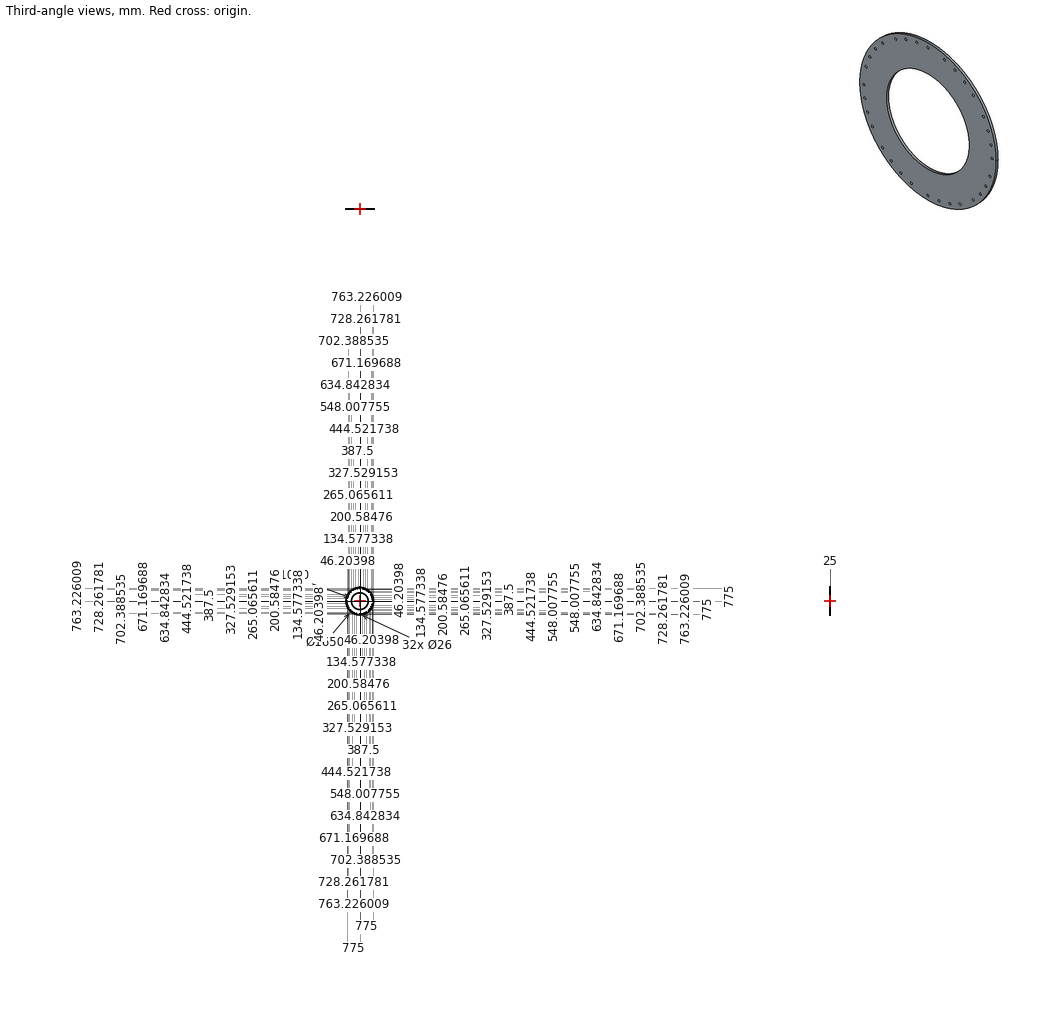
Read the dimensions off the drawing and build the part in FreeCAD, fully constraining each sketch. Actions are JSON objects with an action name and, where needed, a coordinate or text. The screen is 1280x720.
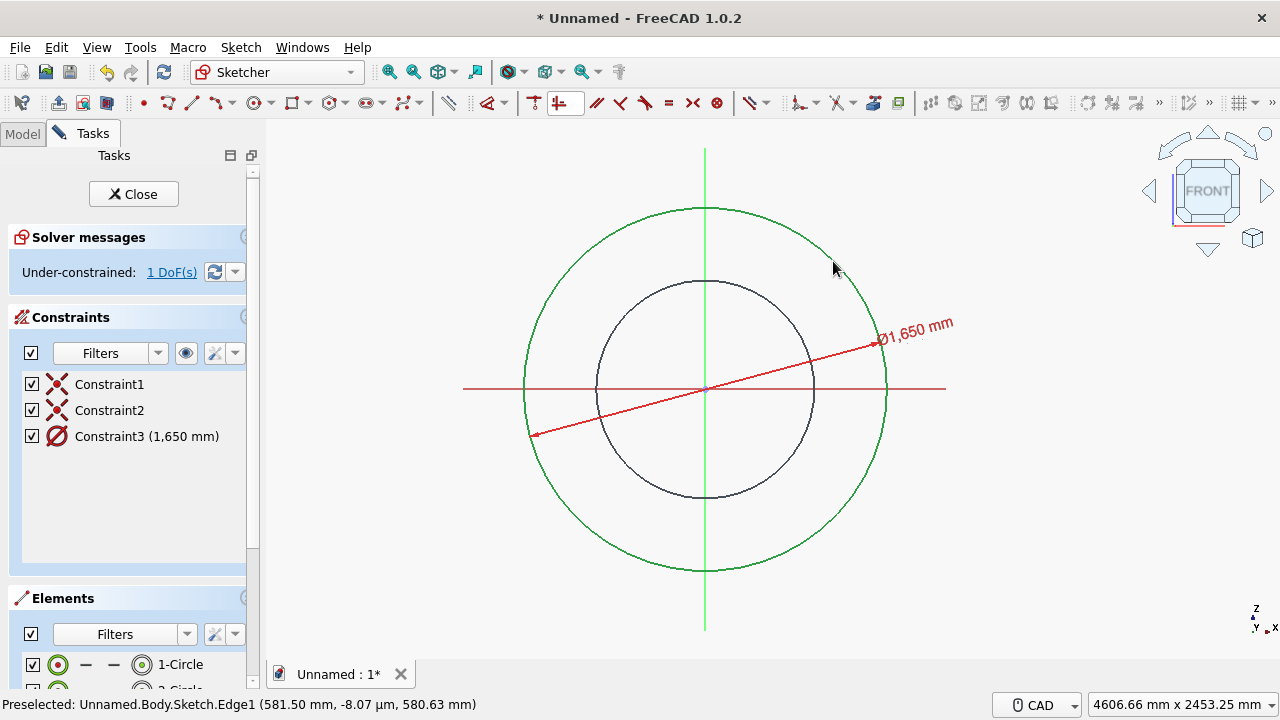
{"action": "left_click", "coordinate": [782, 312]}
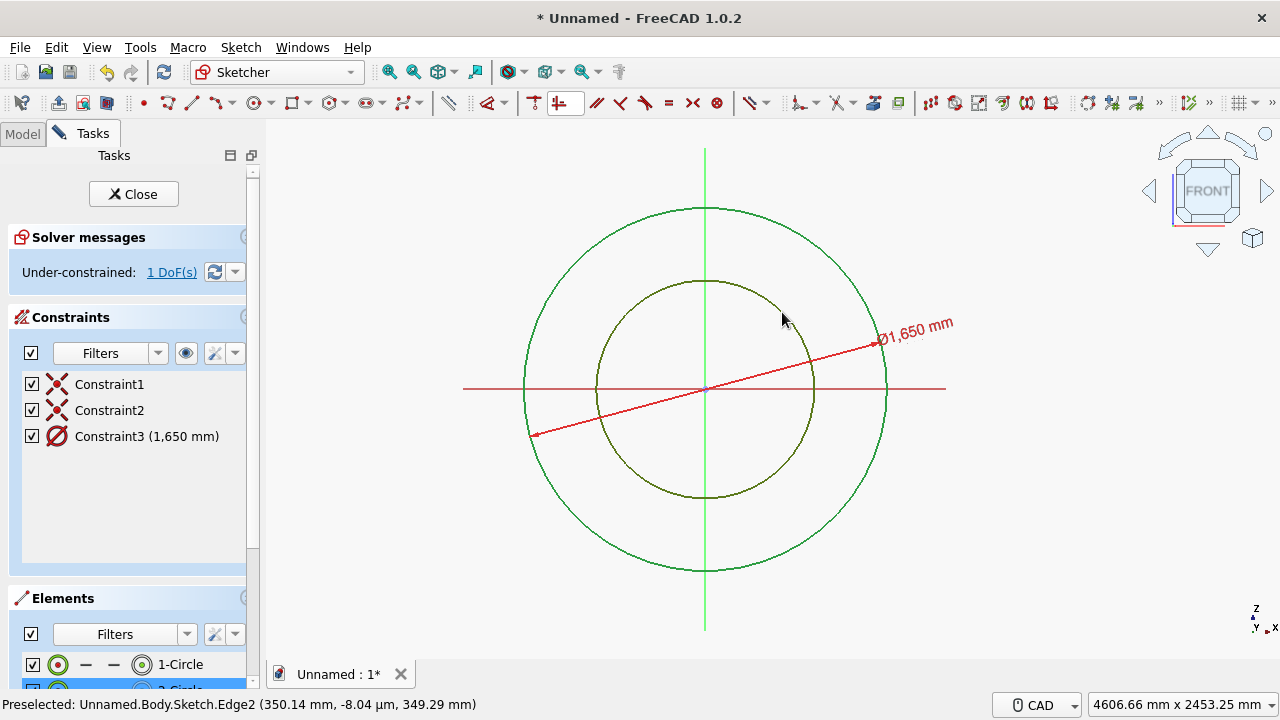
{"action": "key", "text": "k o"}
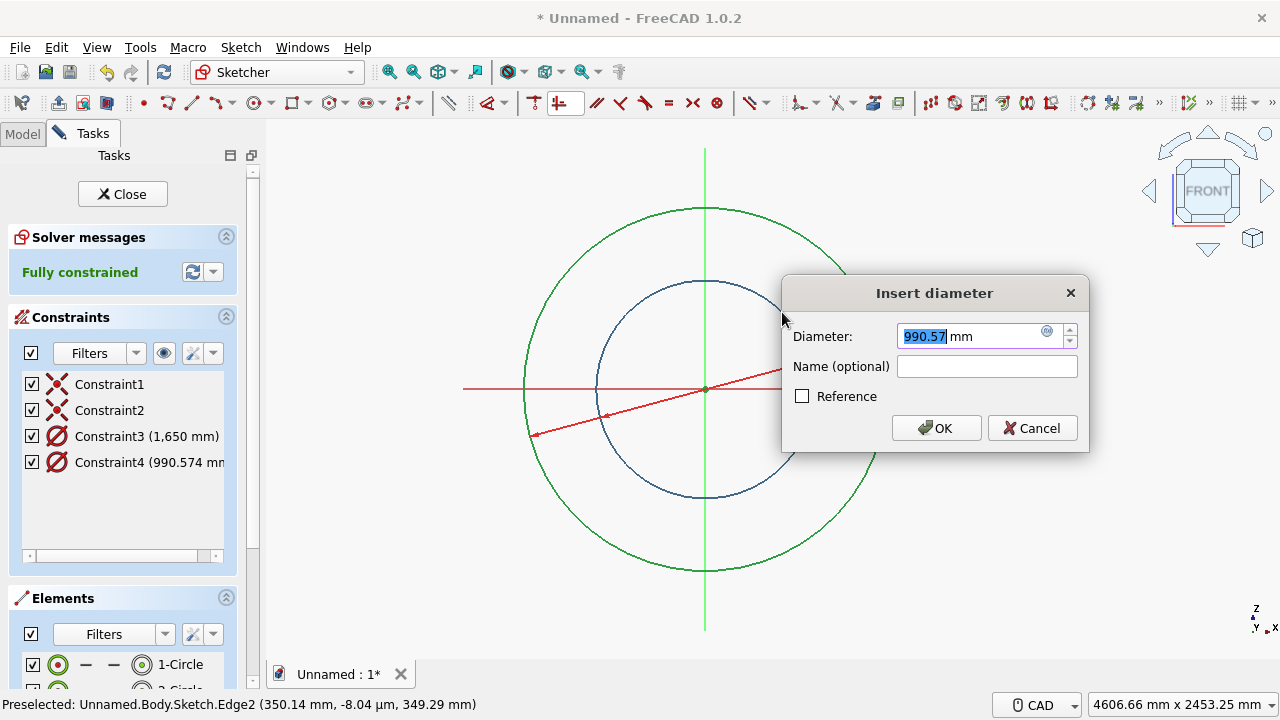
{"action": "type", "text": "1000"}
{"action": "key", "text": "Return"}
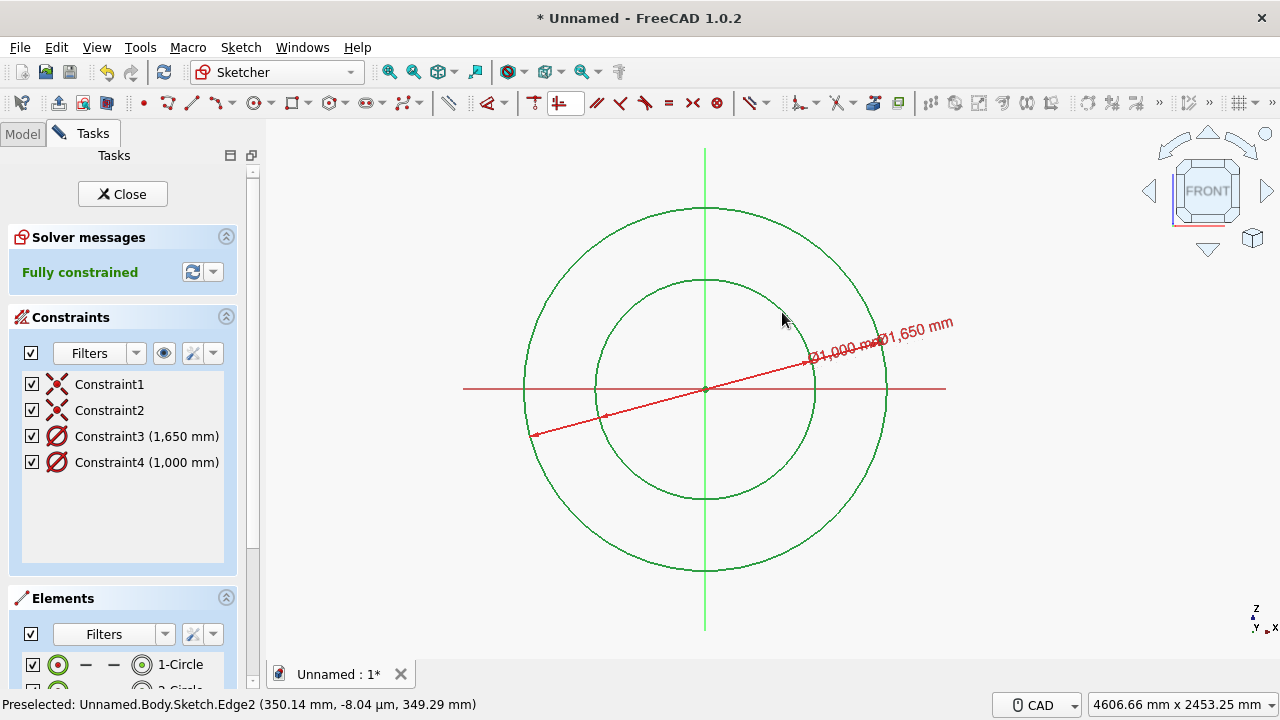
{"action": "left_click", "coordinate": [123, 194]}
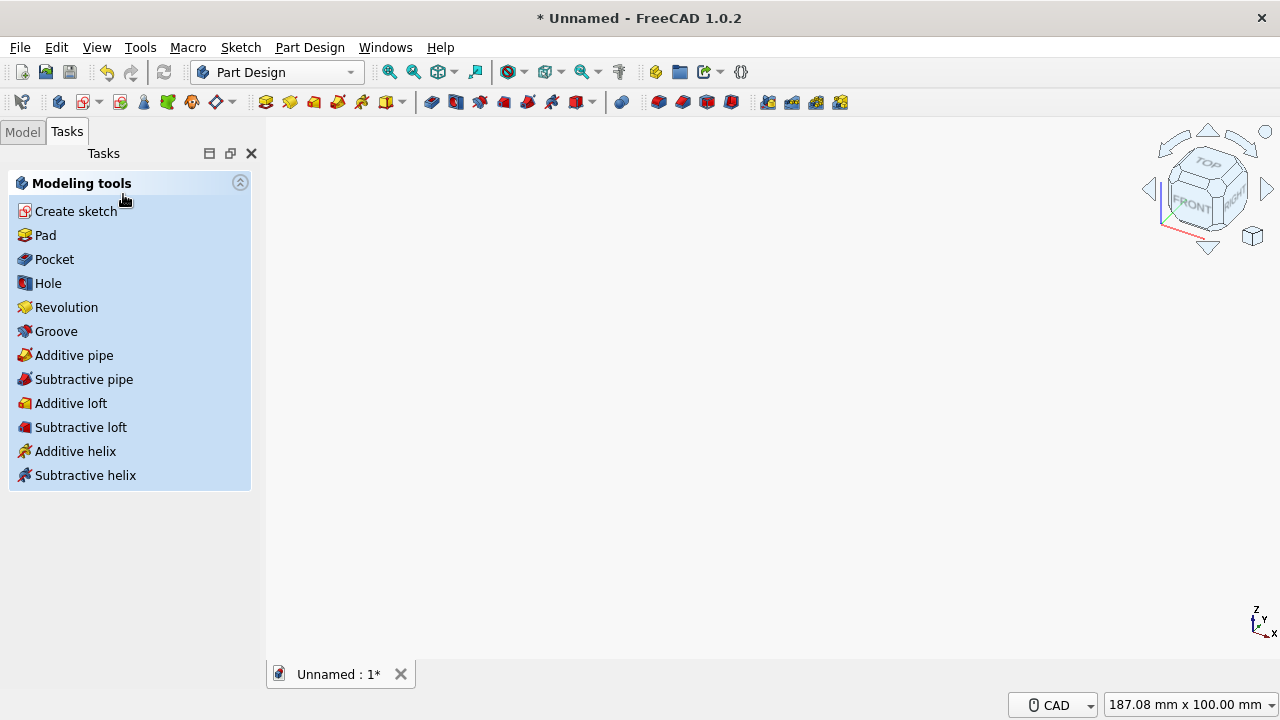
{"action": "left_click", "coordinate": [266, 102]}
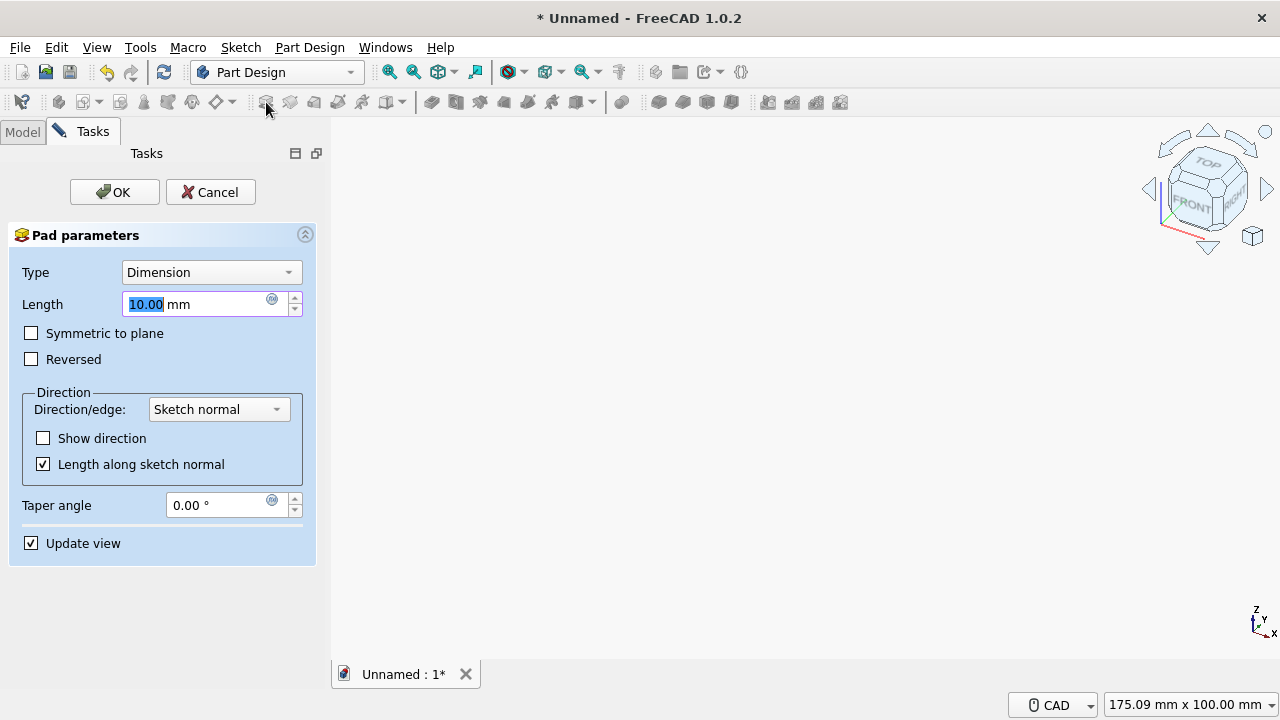
{"action": "type", "text": "25"}
{"action": "key", "text": "Tab"}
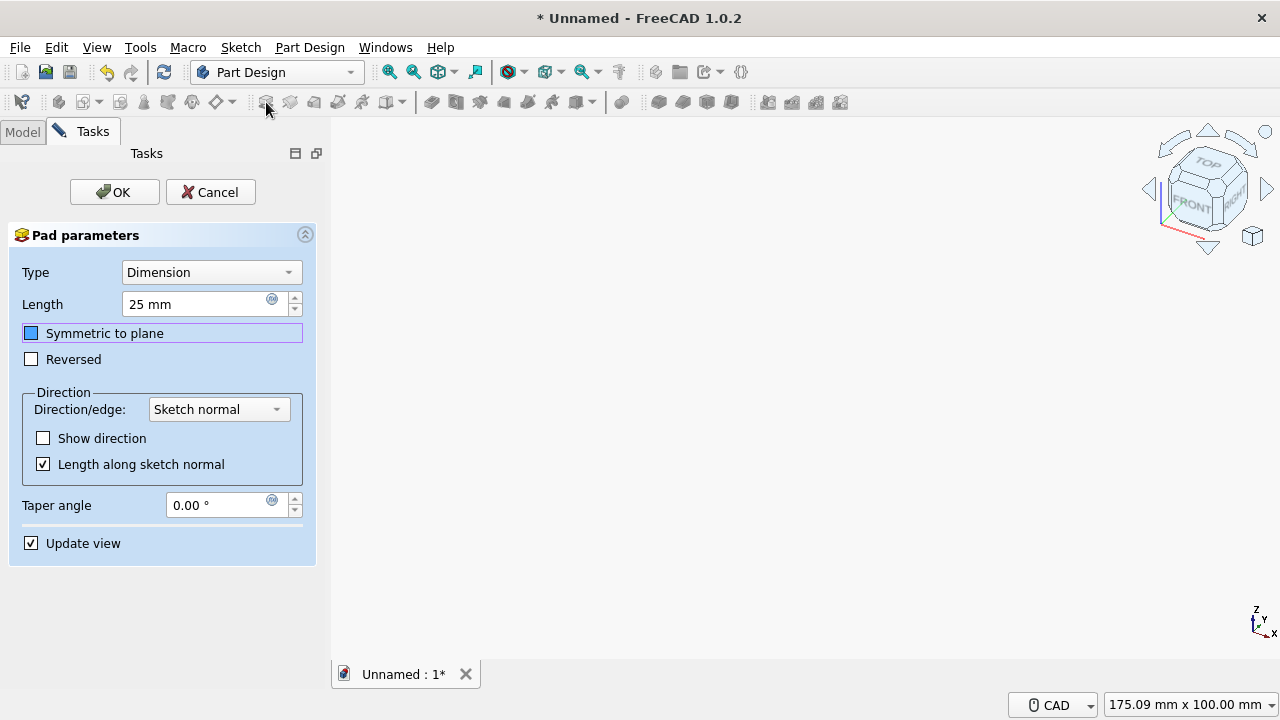
{"action": "left_click", "coordinate": [30, 359]}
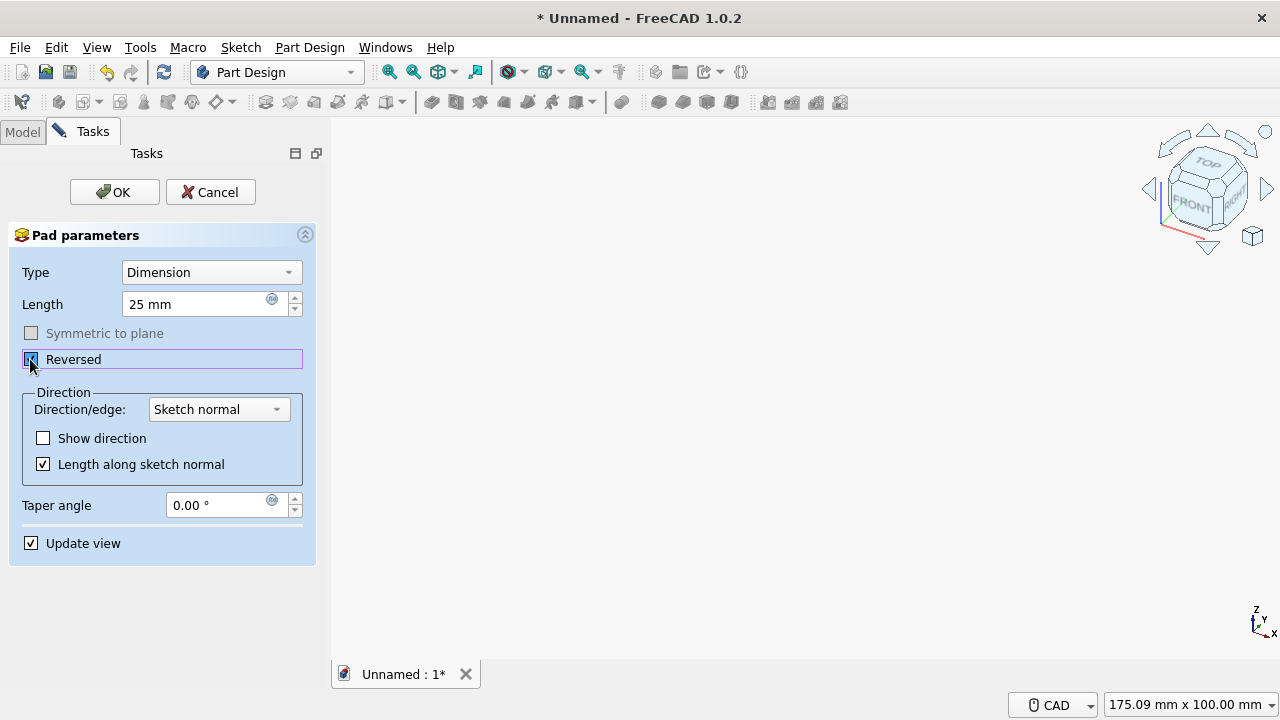
{"action": "left_click", "coordinate": [115, 192]}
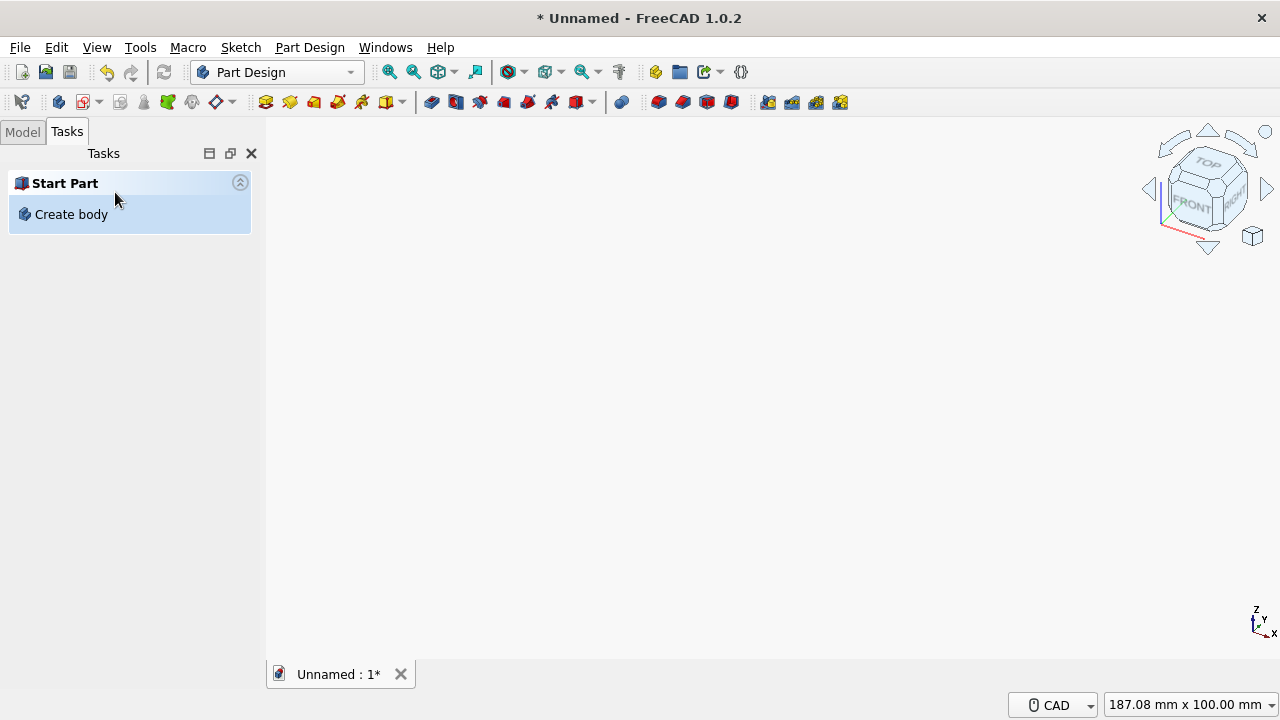
{"action": "left_click", "coordinate": [390, 72]}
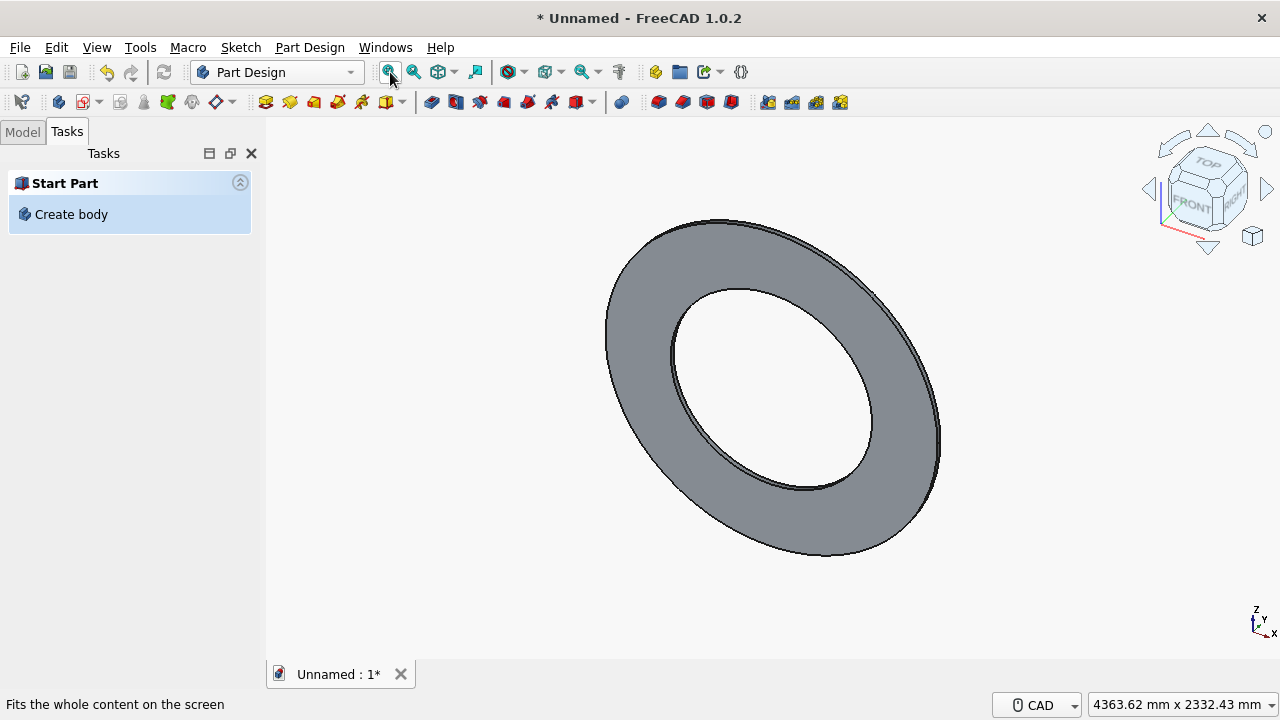
{"action": "key", "text": "4"}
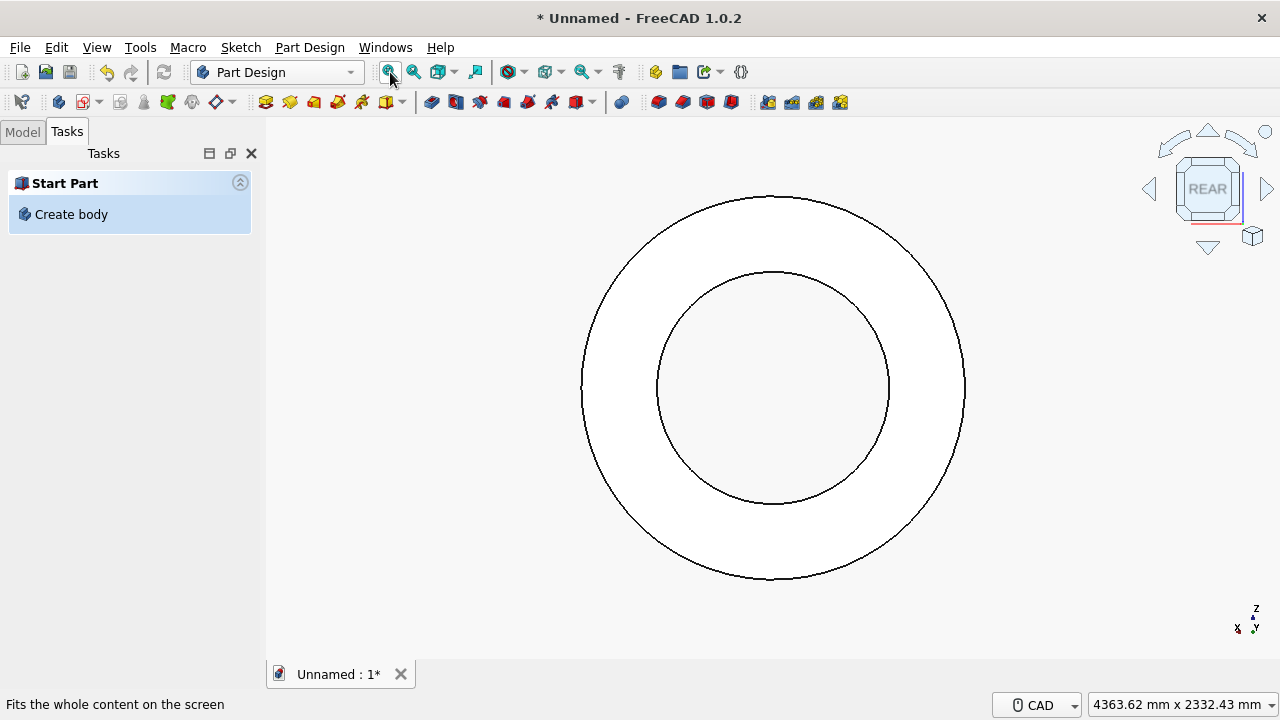
{"action": "left_click", "coordinate": [664, 277]}